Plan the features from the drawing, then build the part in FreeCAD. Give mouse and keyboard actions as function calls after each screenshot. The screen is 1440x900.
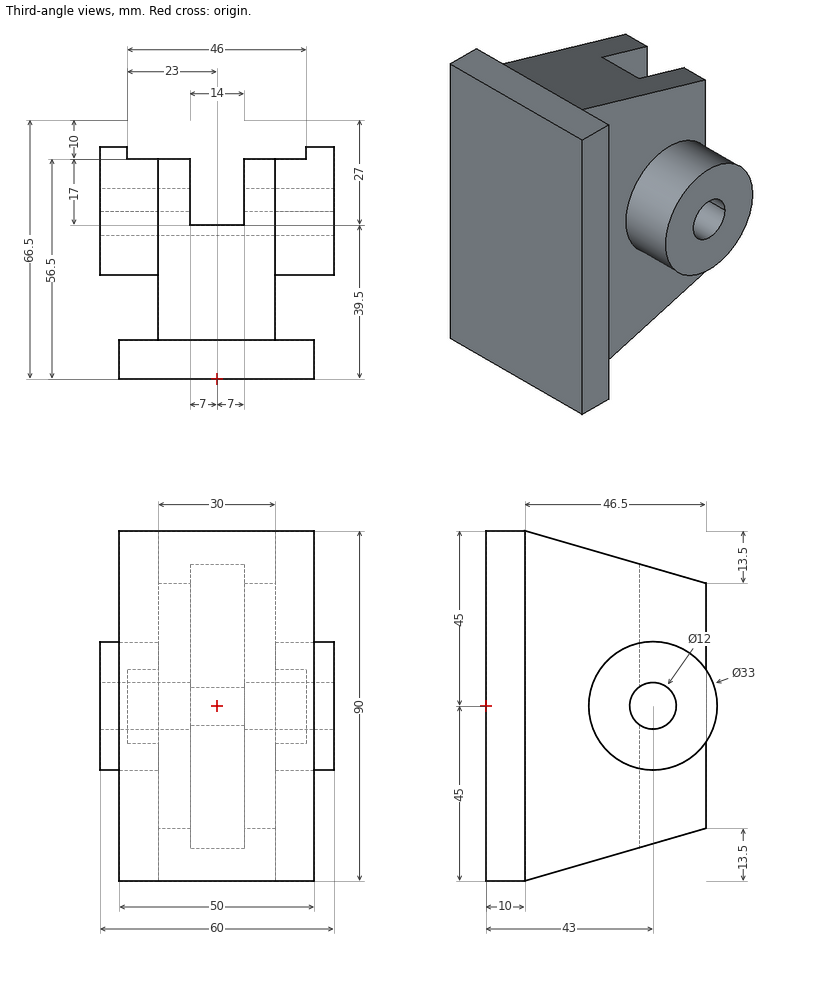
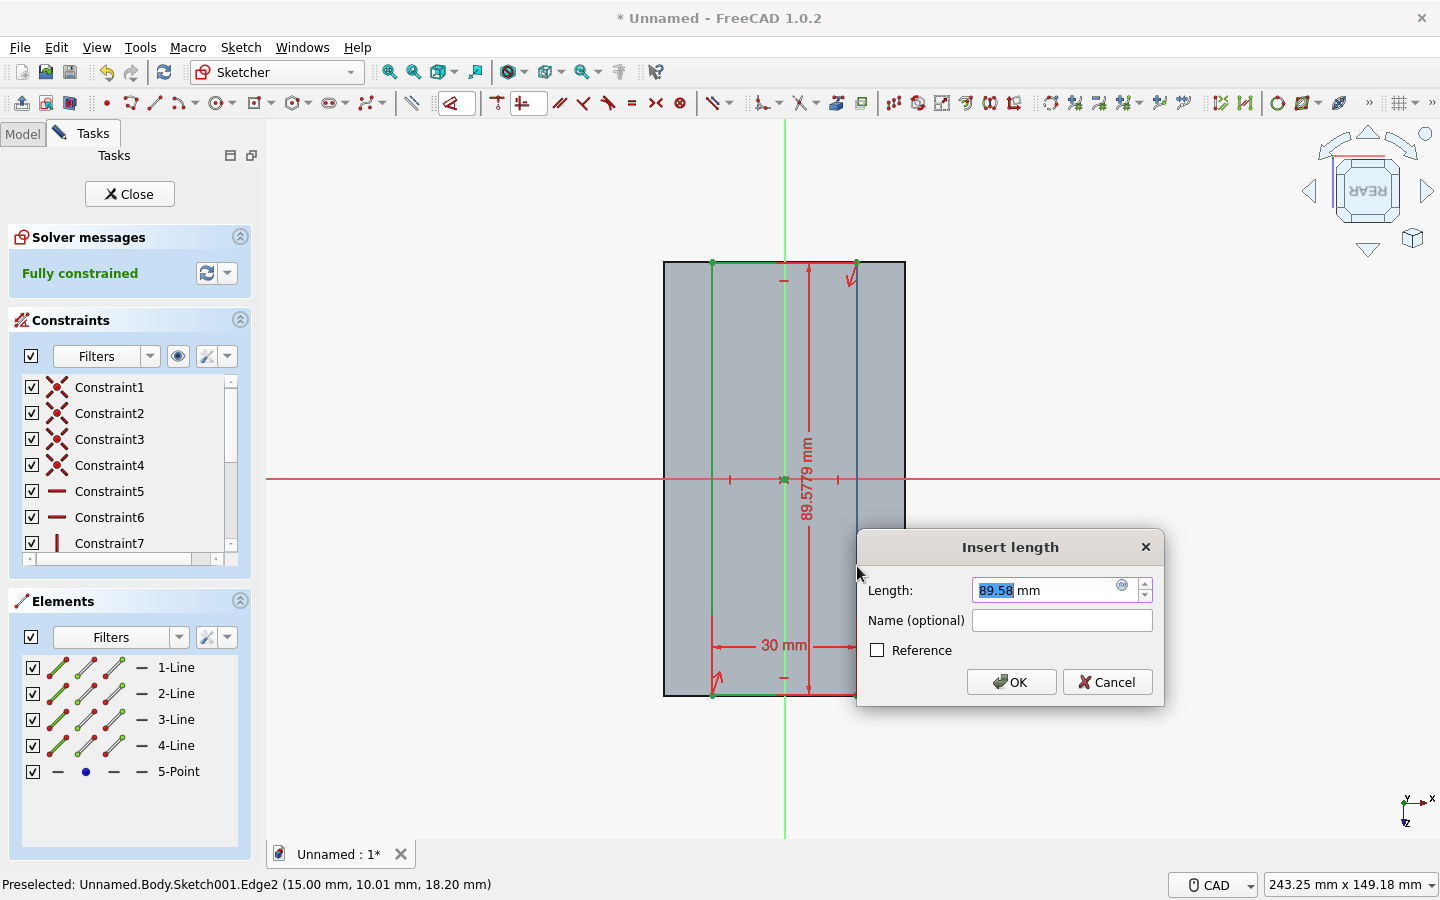
text(90)
key(Return)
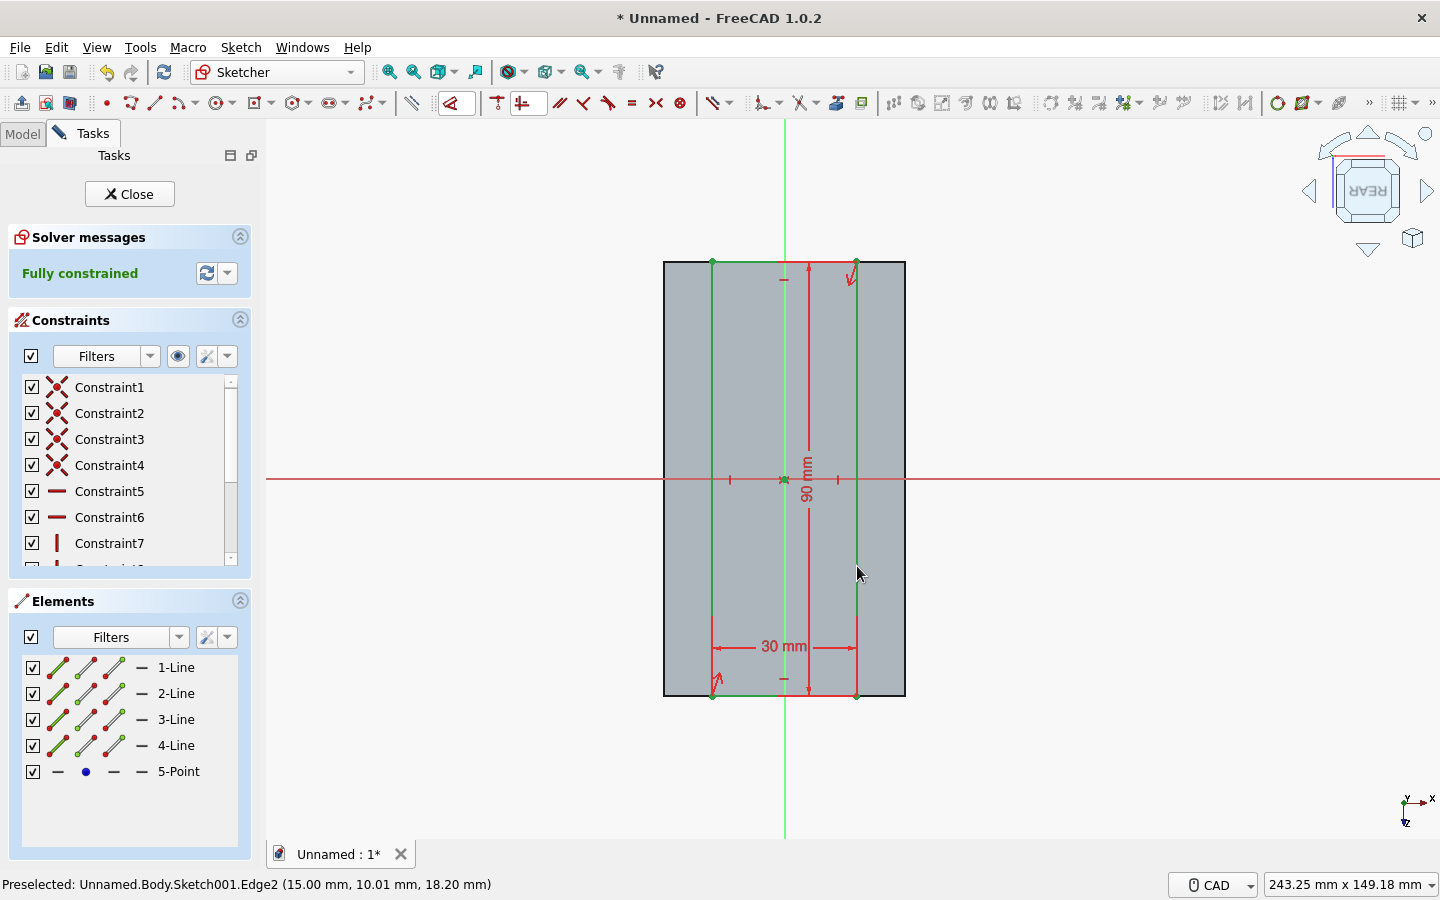
click(130, 194)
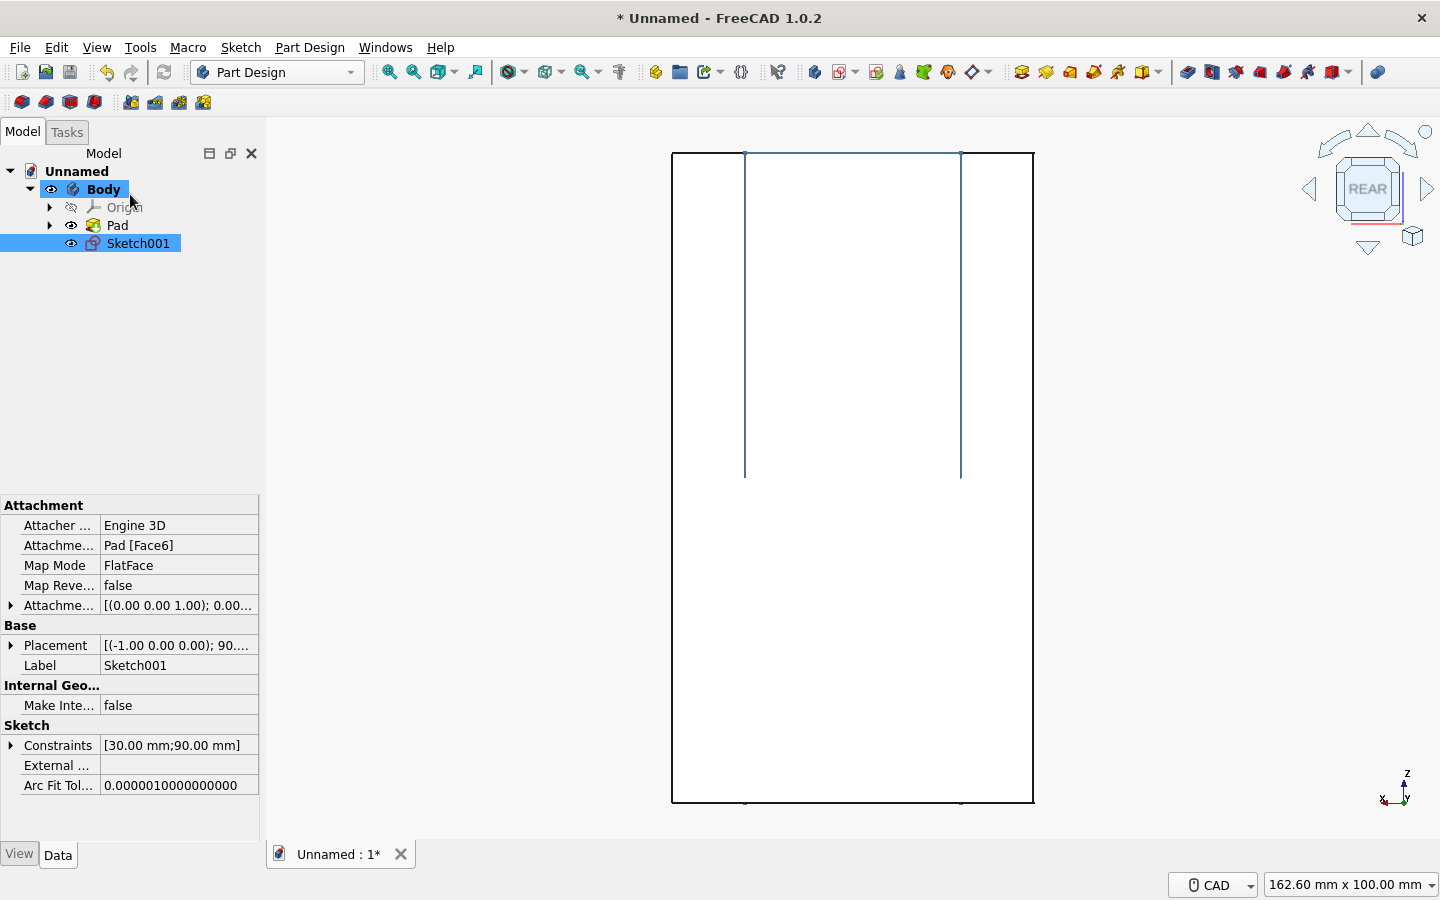
click(1022, 72)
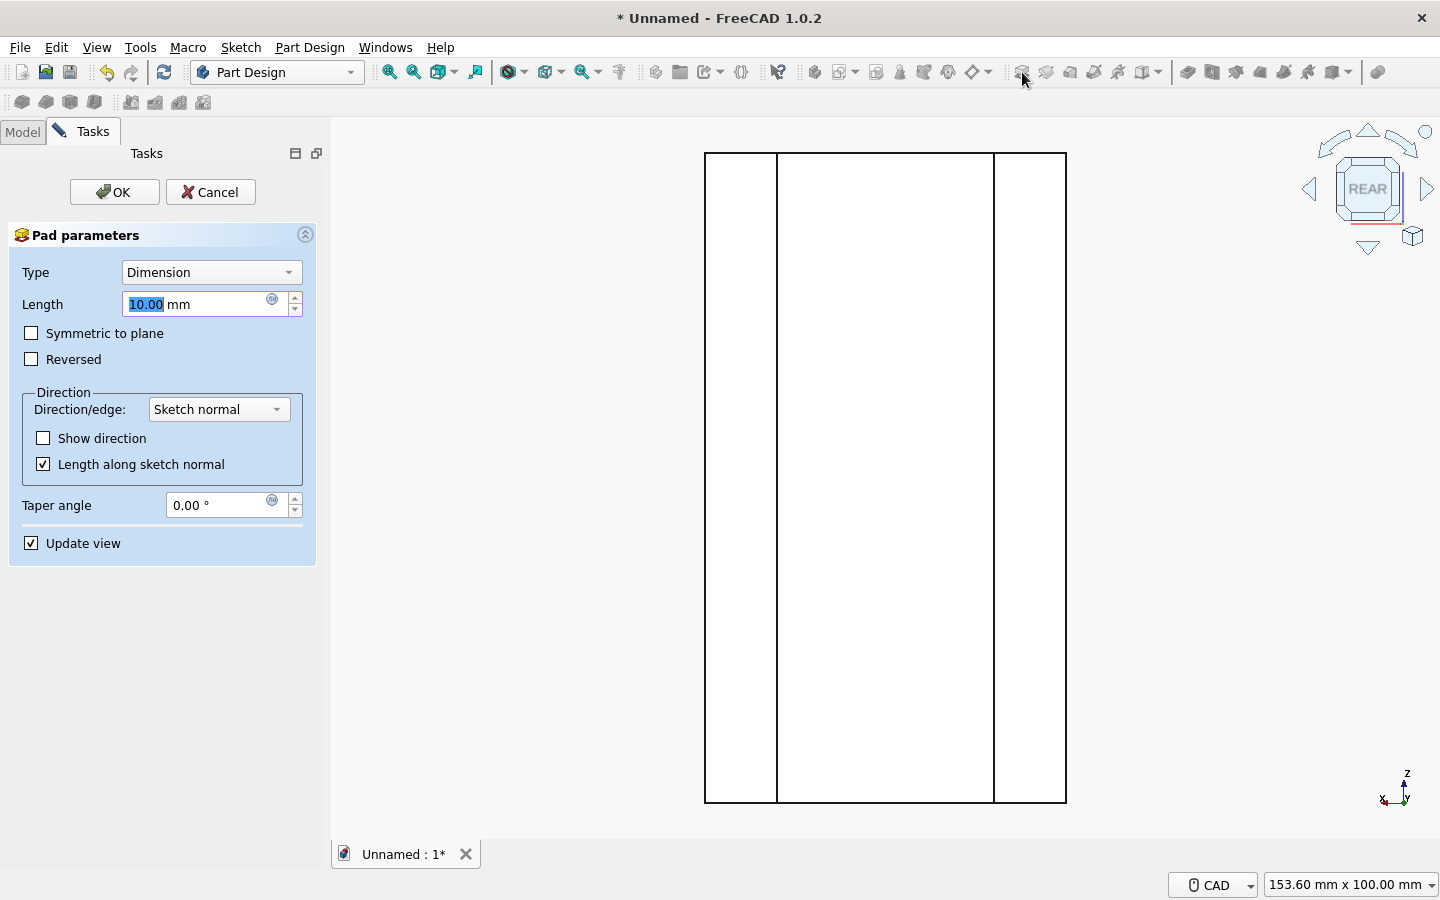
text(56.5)
key(Tab)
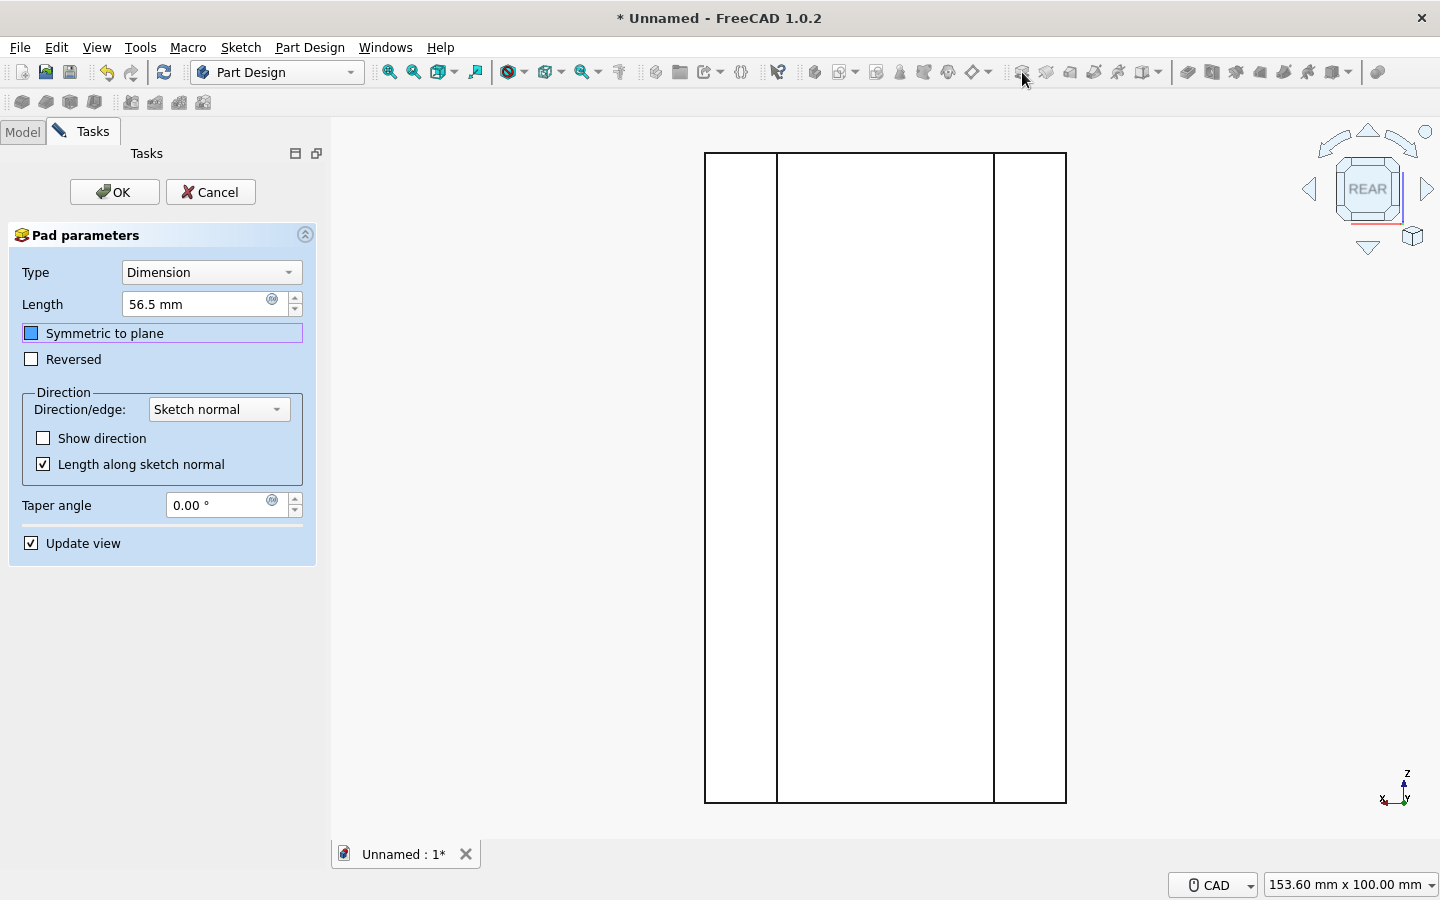
click(115, 192)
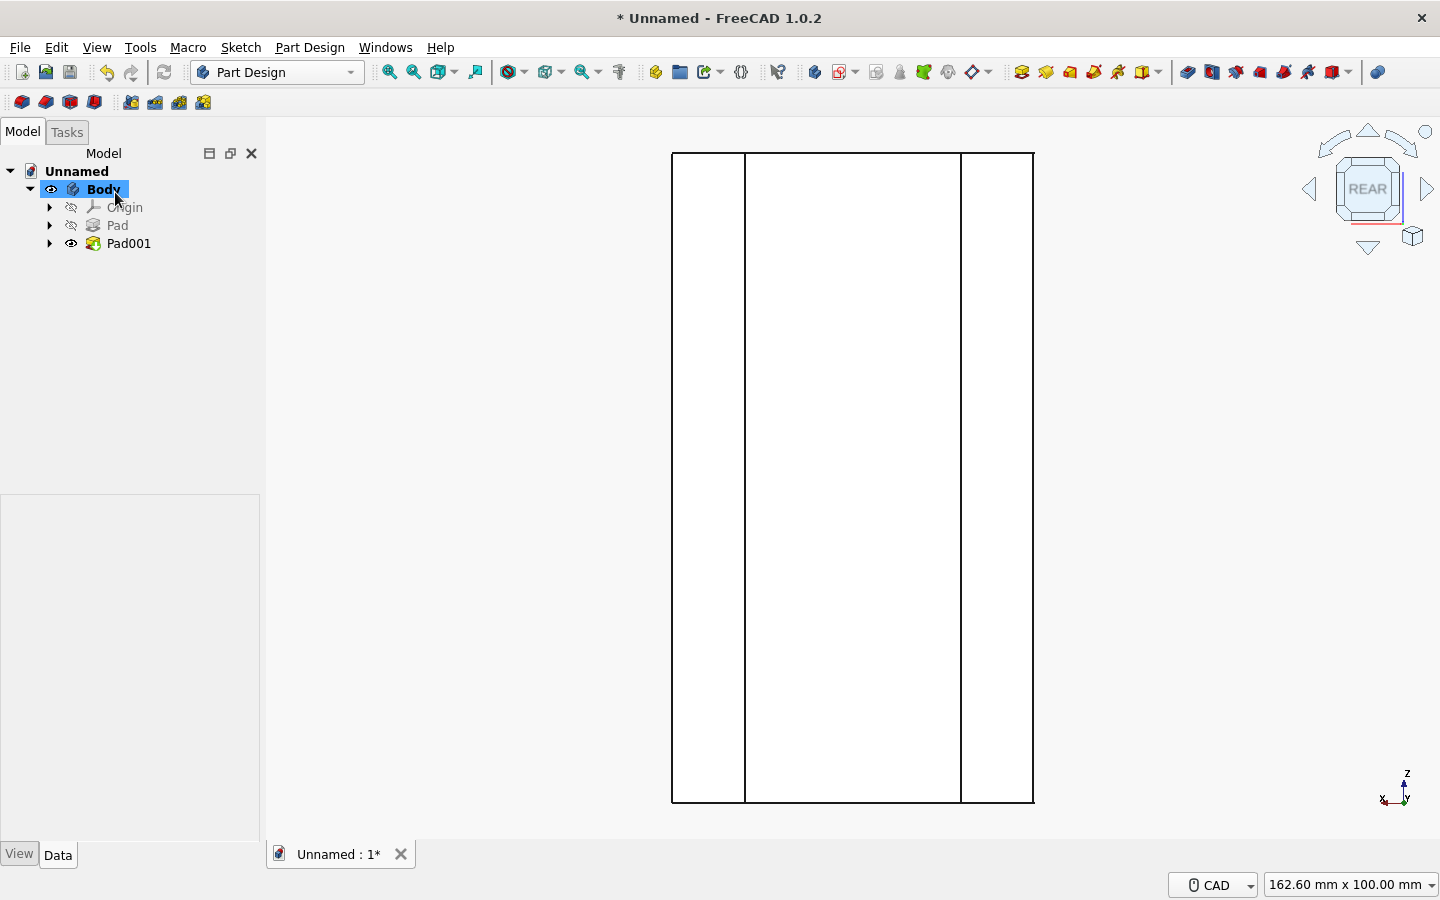
key(0)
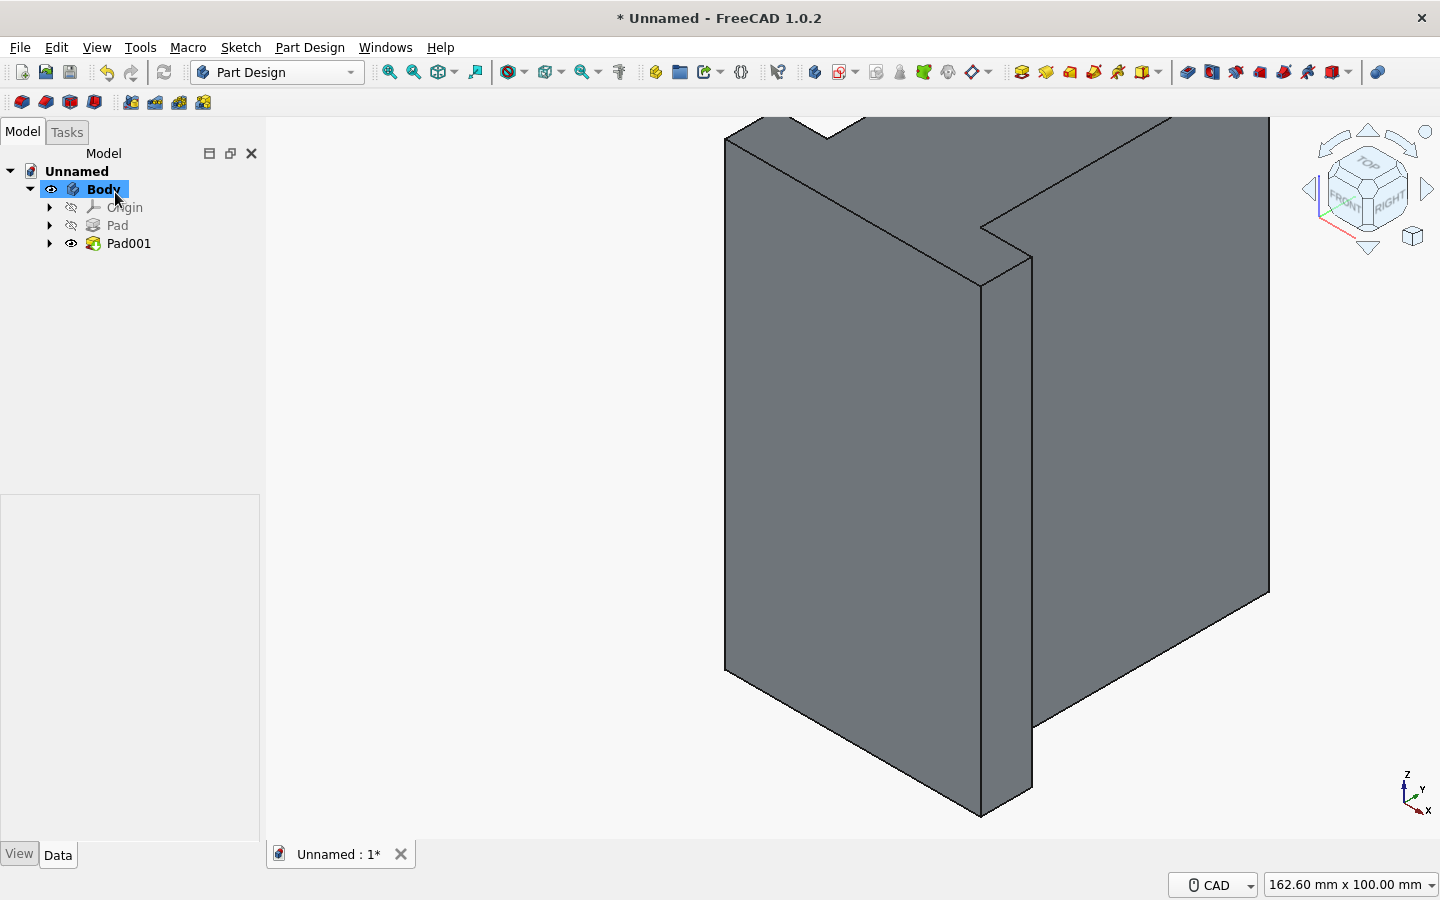
click(390, 72)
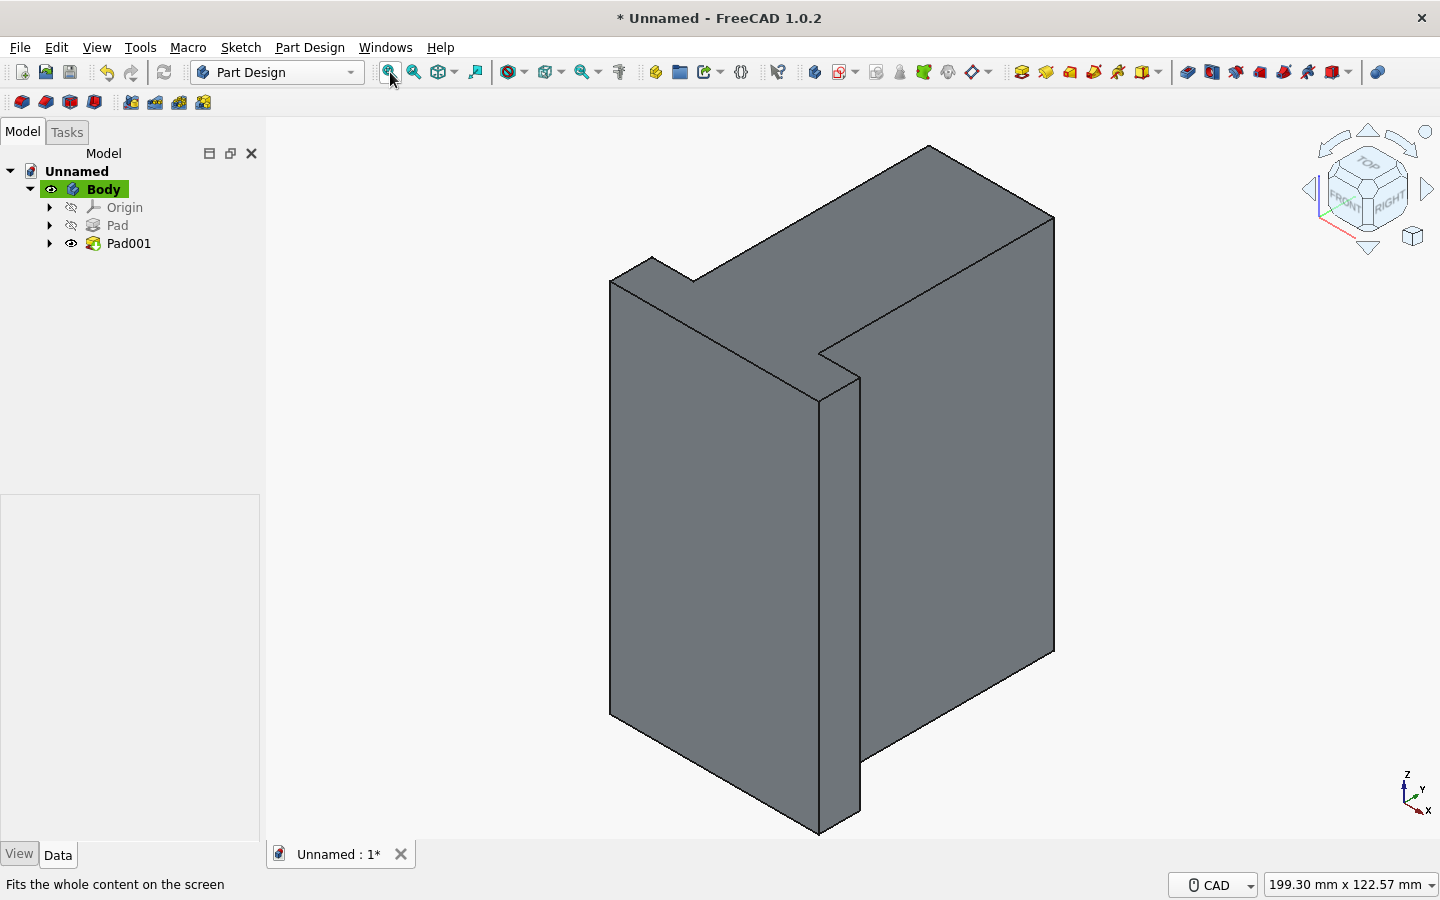
click(893, 238)